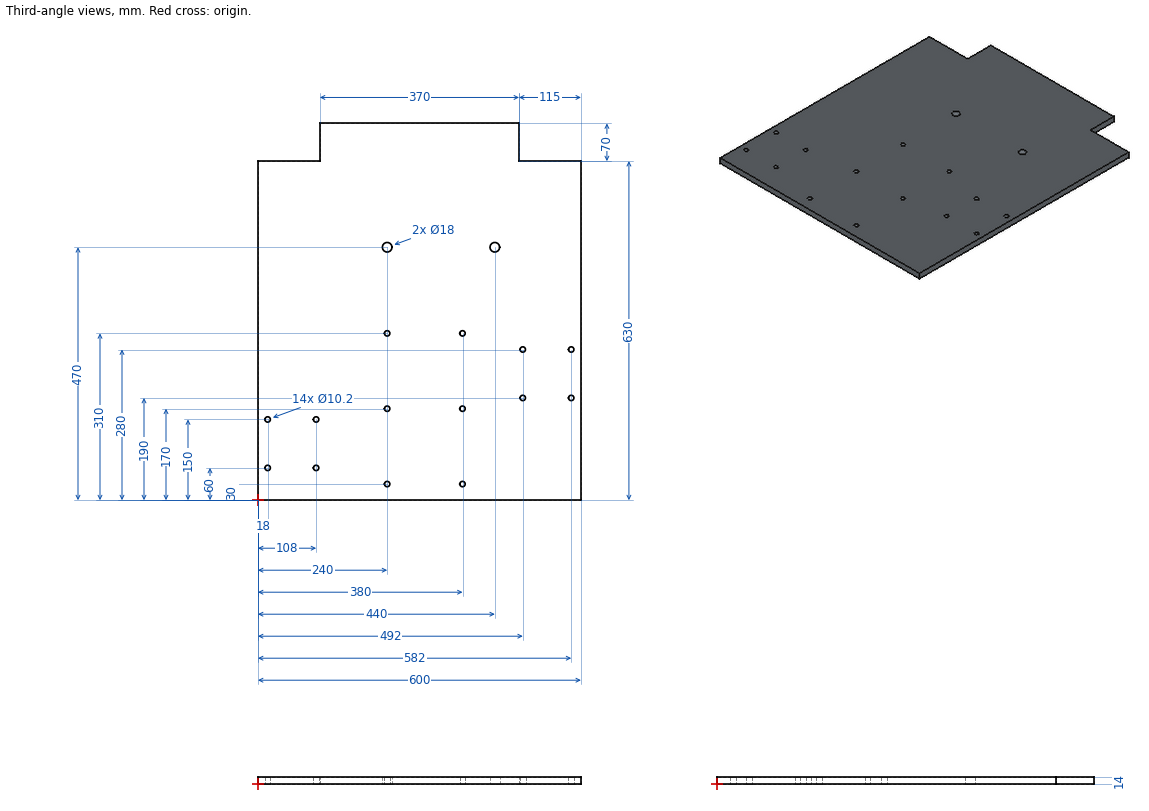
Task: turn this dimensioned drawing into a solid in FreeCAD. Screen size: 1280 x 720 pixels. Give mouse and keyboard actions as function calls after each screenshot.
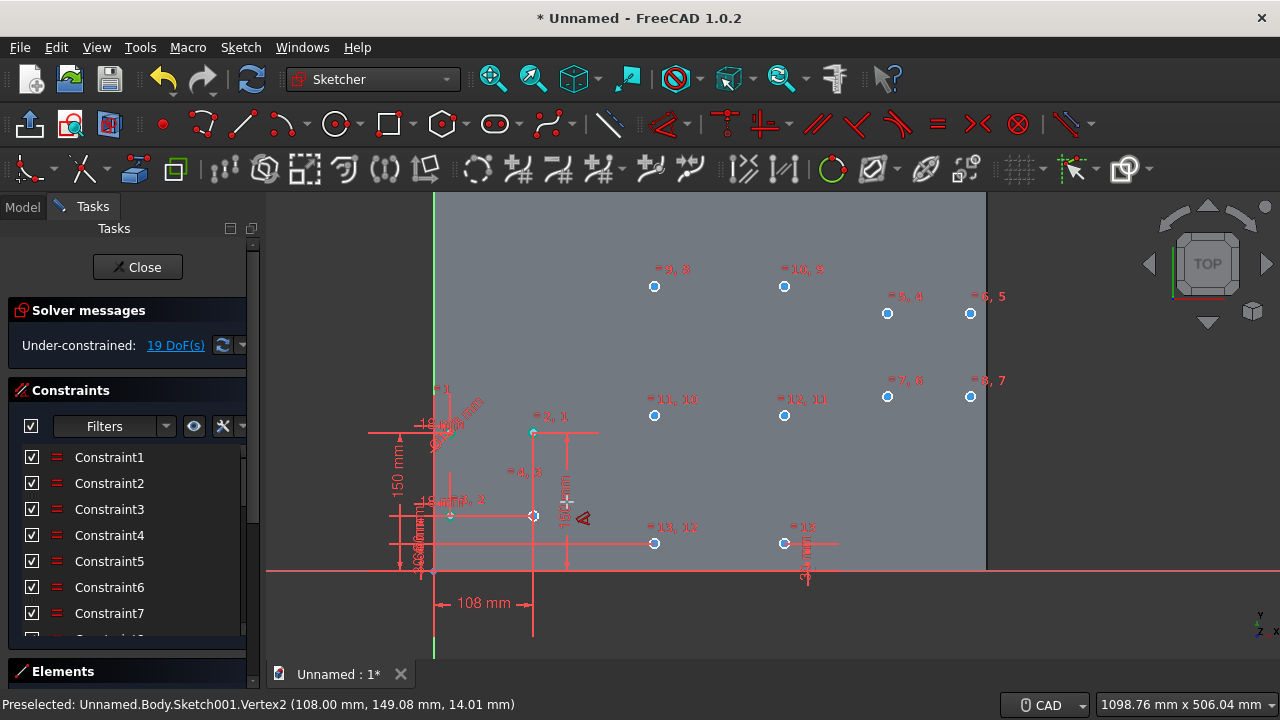
click(534, 516)
click(484, 482)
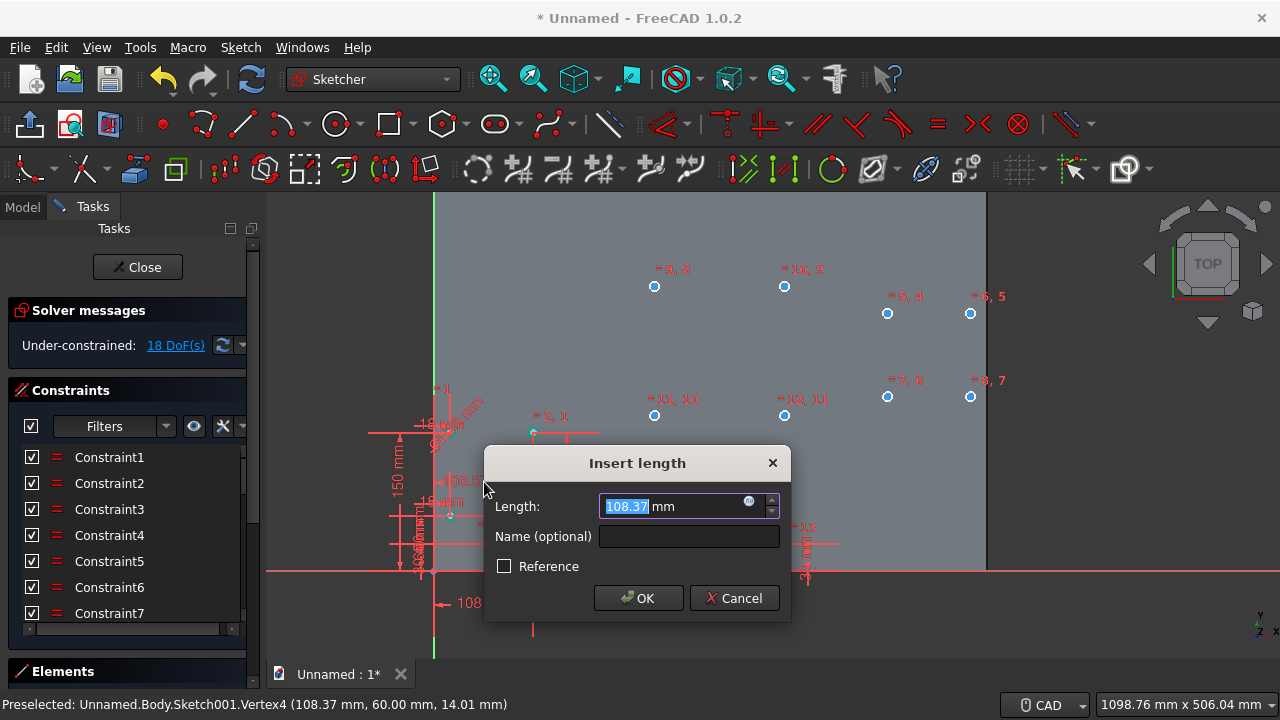
text(108)
key(Return)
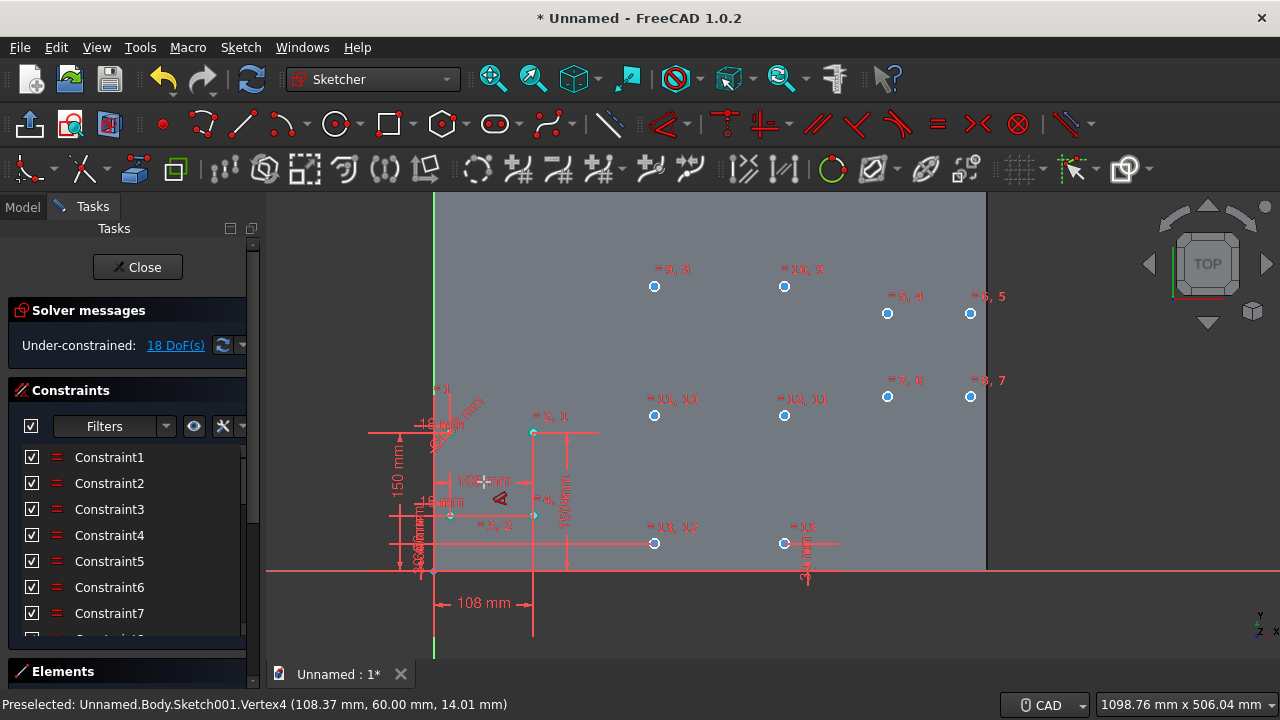
click(888, 313)
click(661, 605)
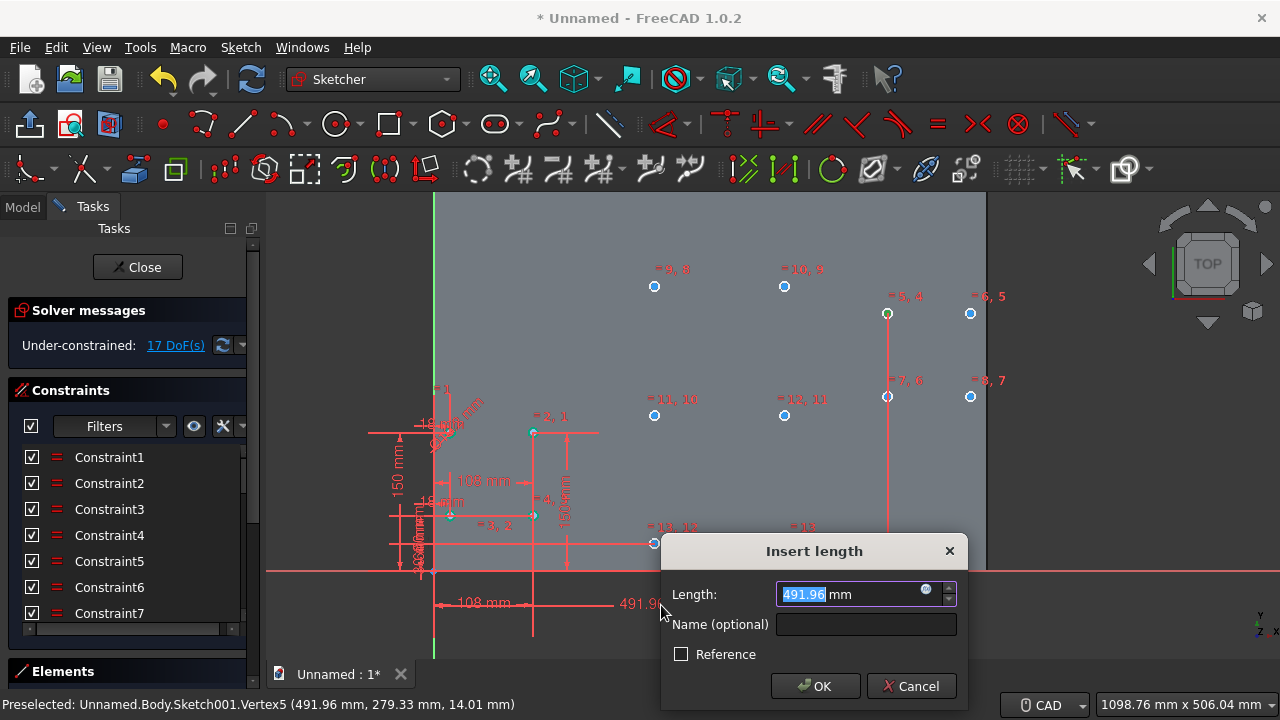
text(492)
key(Return)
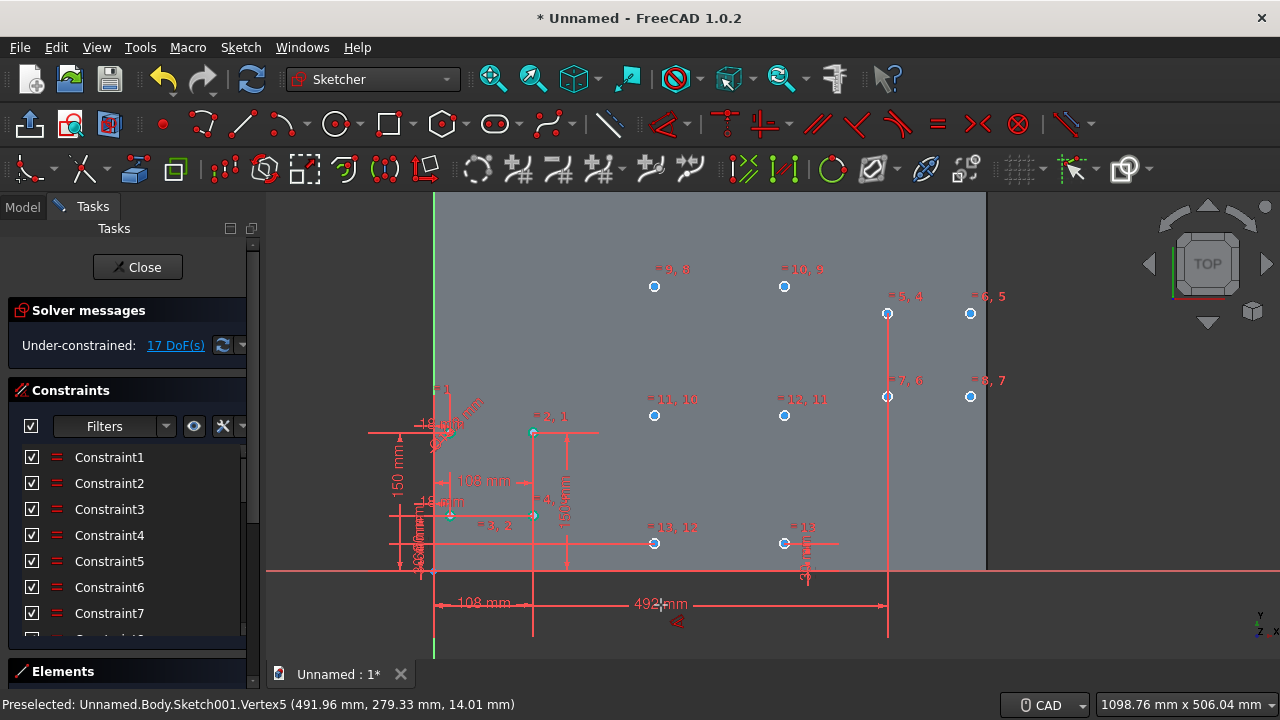
click(888, 313)
click(400, 383)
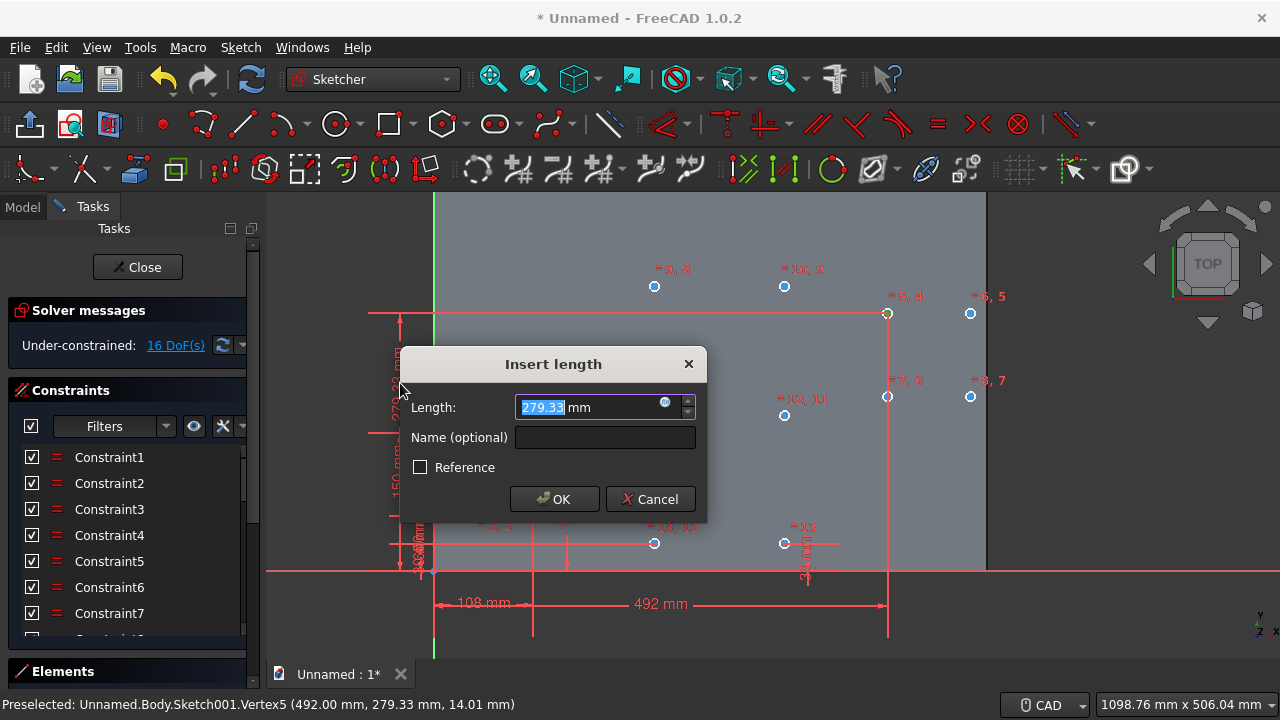
text(280)
key(Return)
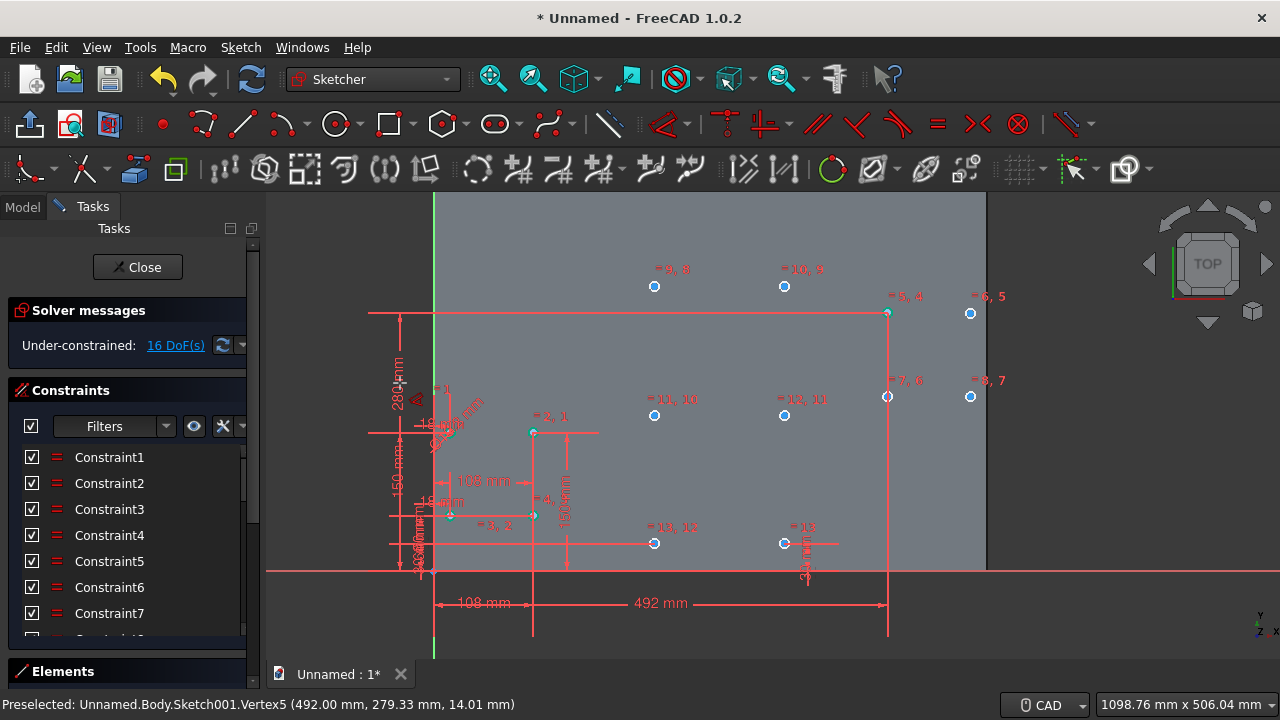
click(971, 313)
click(579, 605)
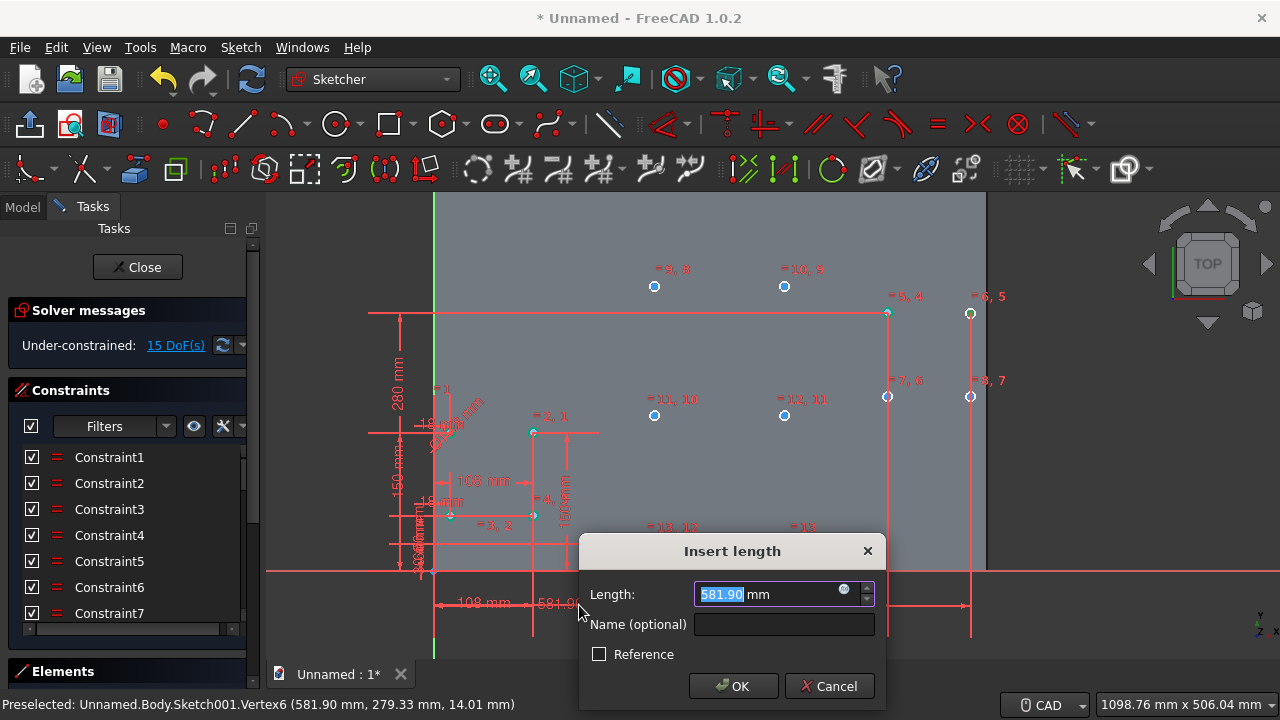
text(582)
key(Return)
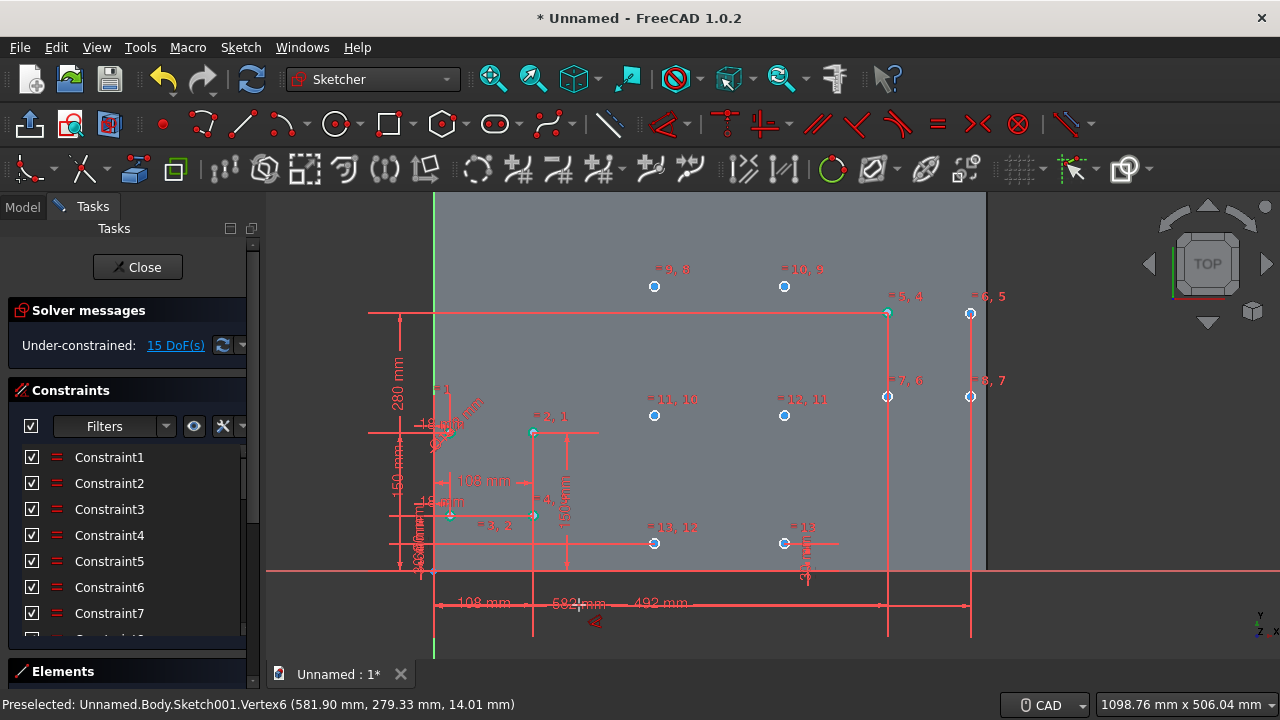
click(971, 313)
click(400, 352)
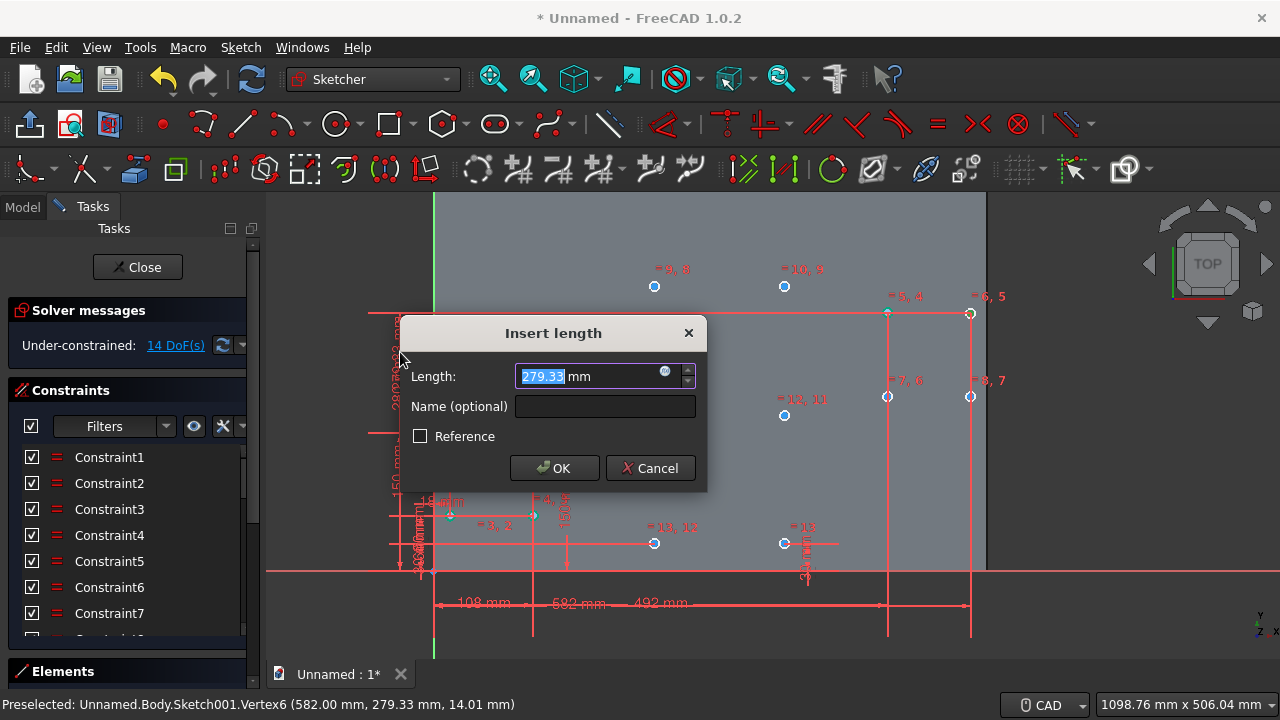
text(280)
key(Return)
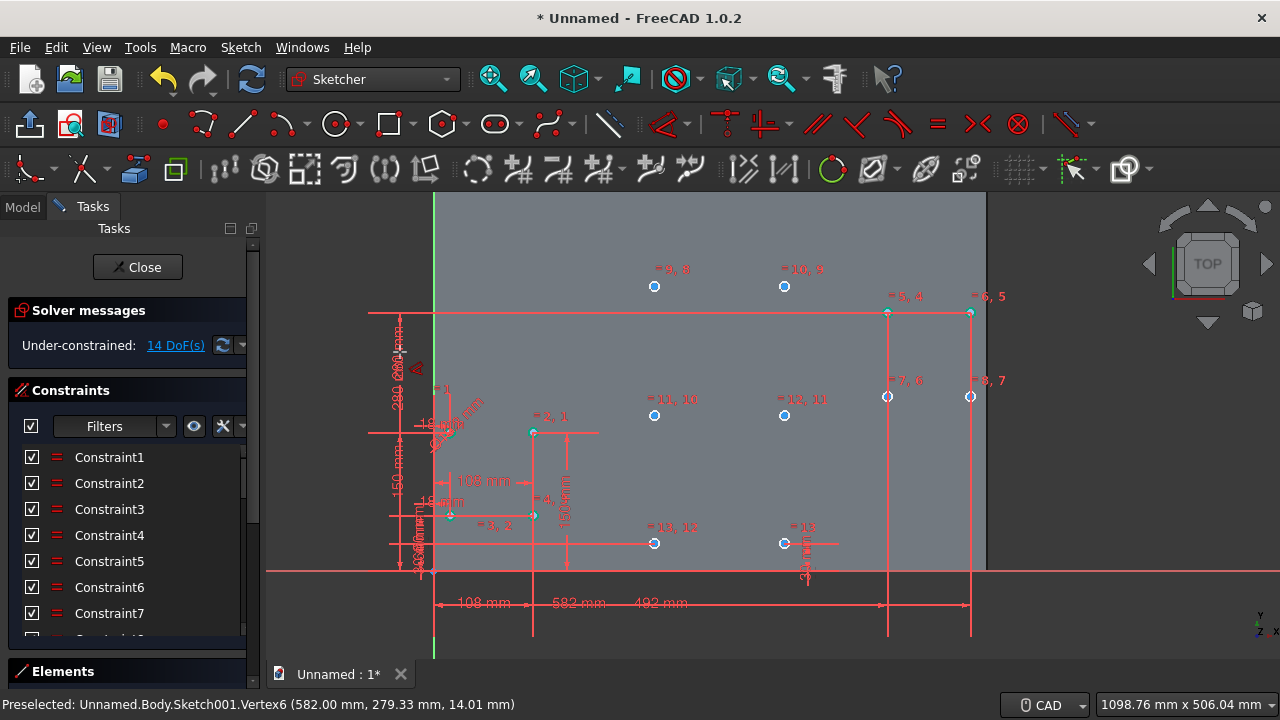
click(888, 397)
click(765, 605)